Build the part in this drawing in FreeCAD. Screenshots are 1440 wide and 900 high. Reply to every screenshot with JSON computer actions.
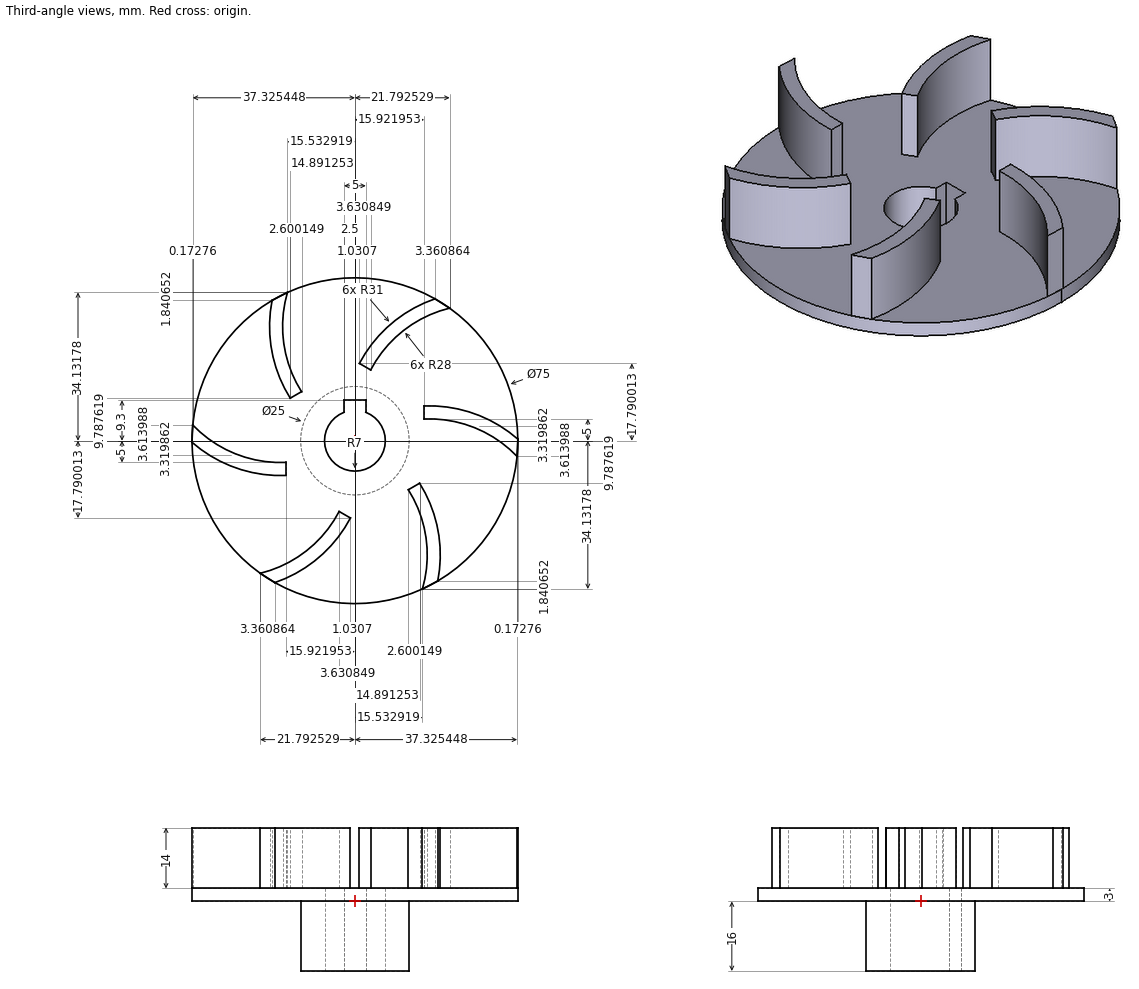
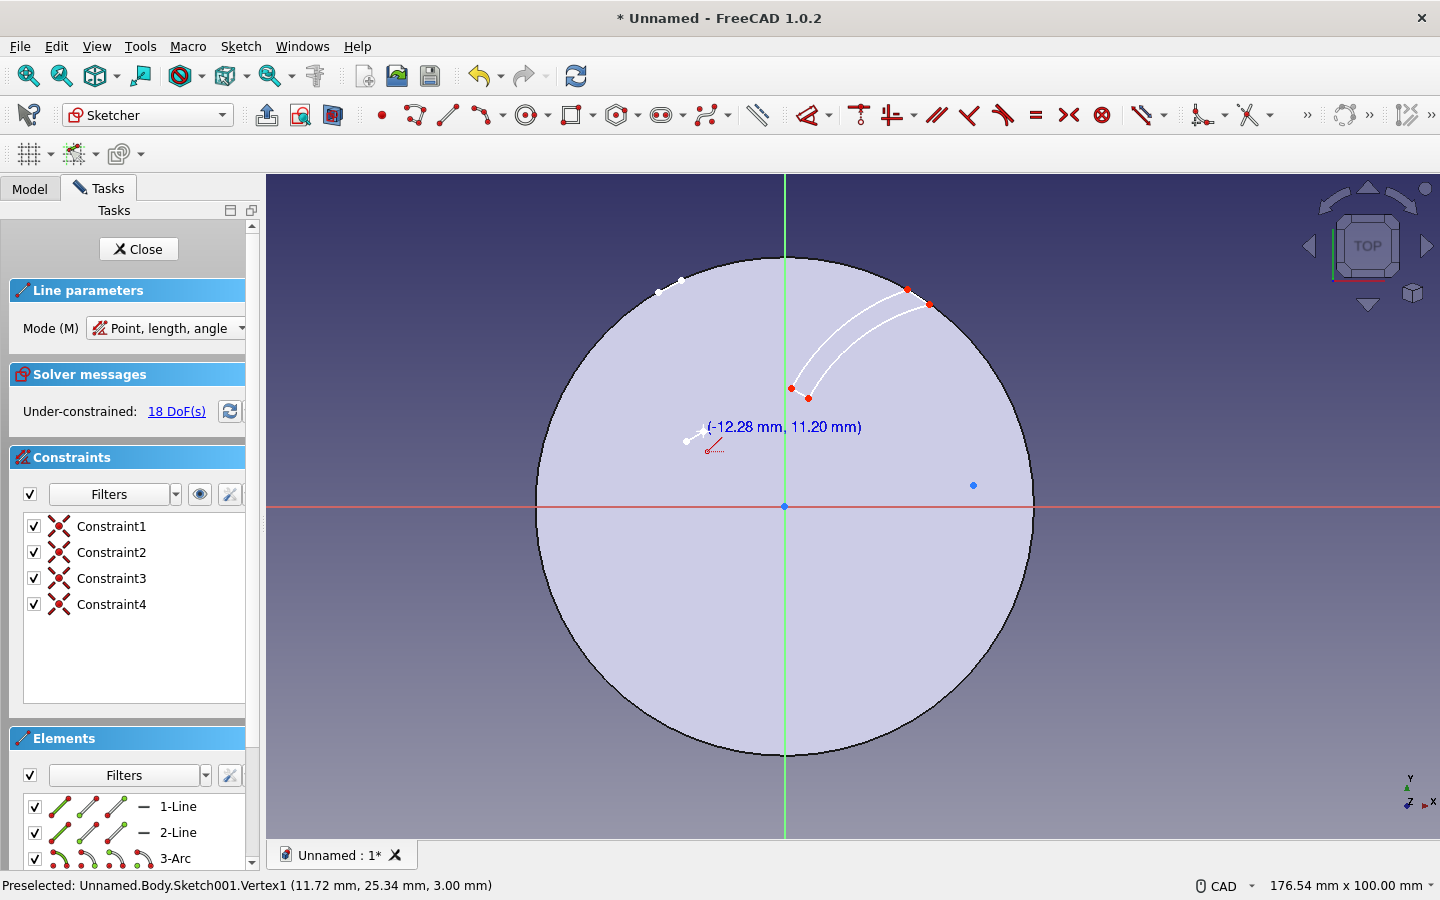
{"action": "left_click", "coordinate": [480, 116]}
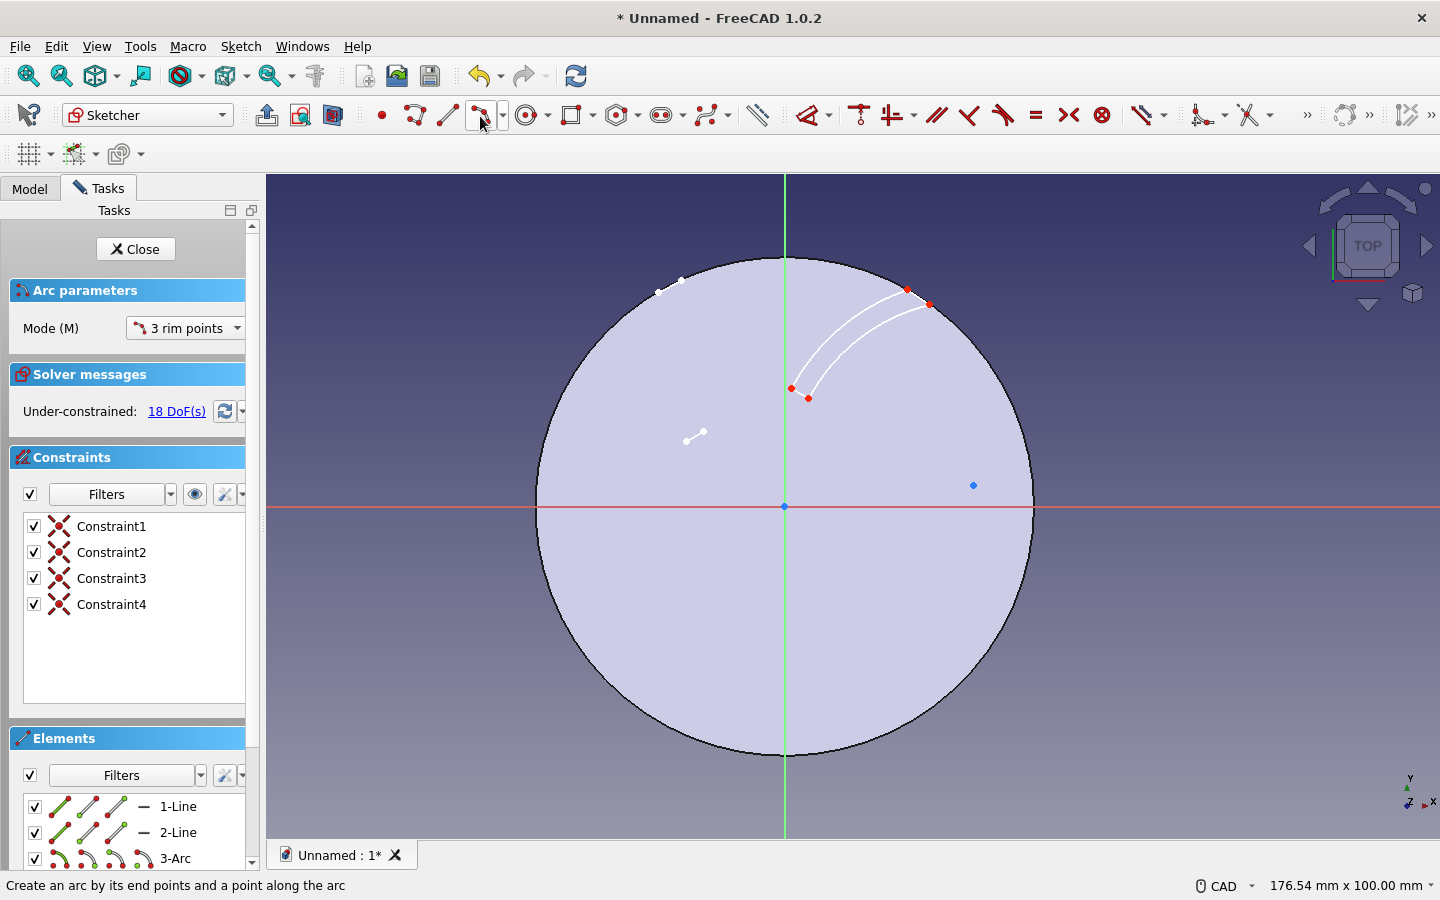
{"action": "left_click", "coordinate": [658, 293]}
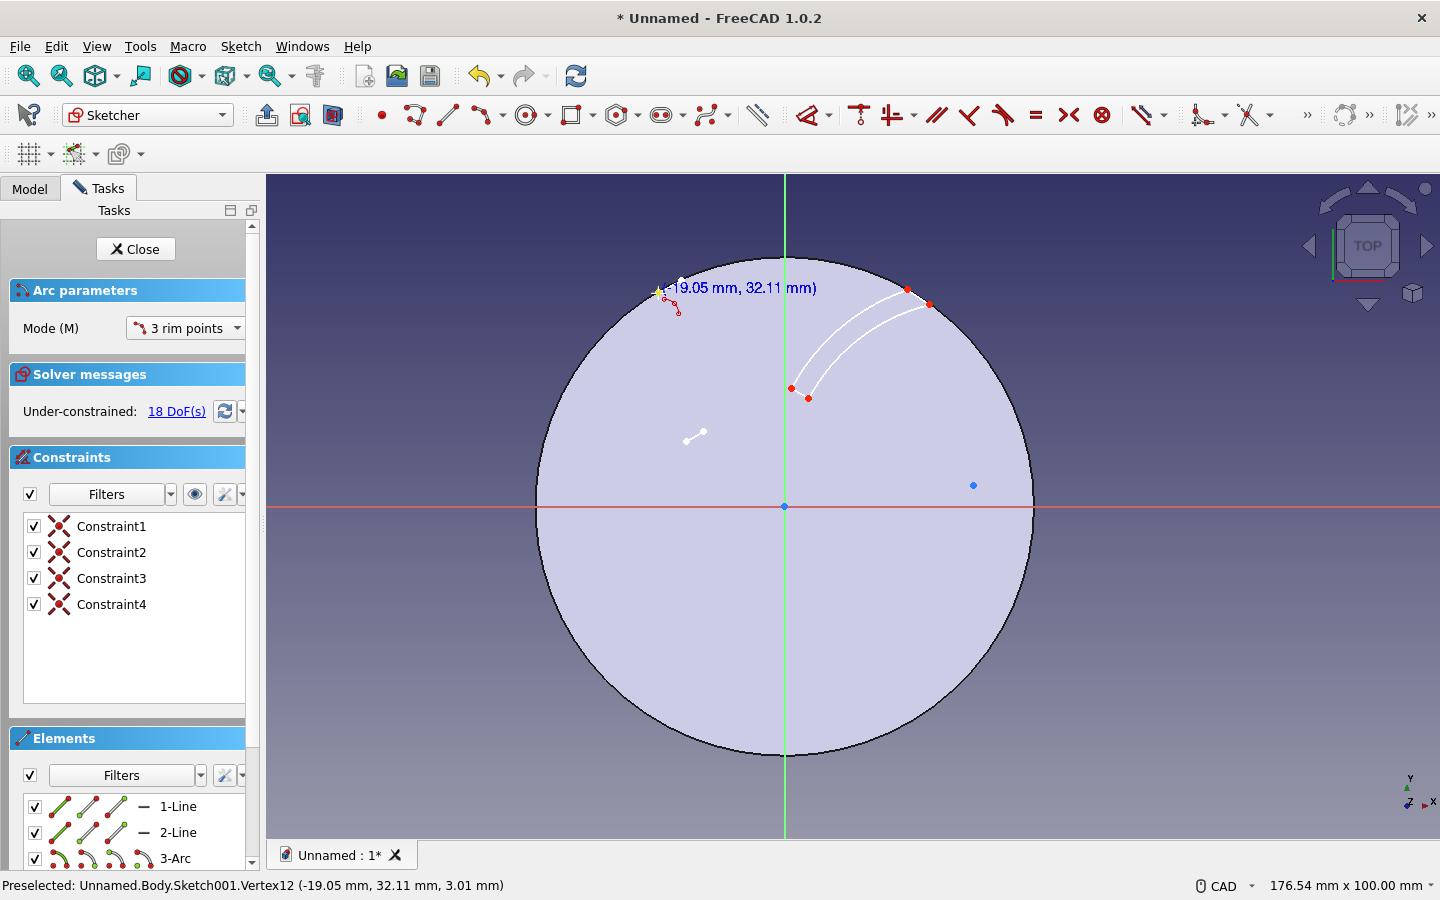
{"action": "scroll", "coordinate": [686, 441], "scroll_direction": "up", "scroll_amount": 3}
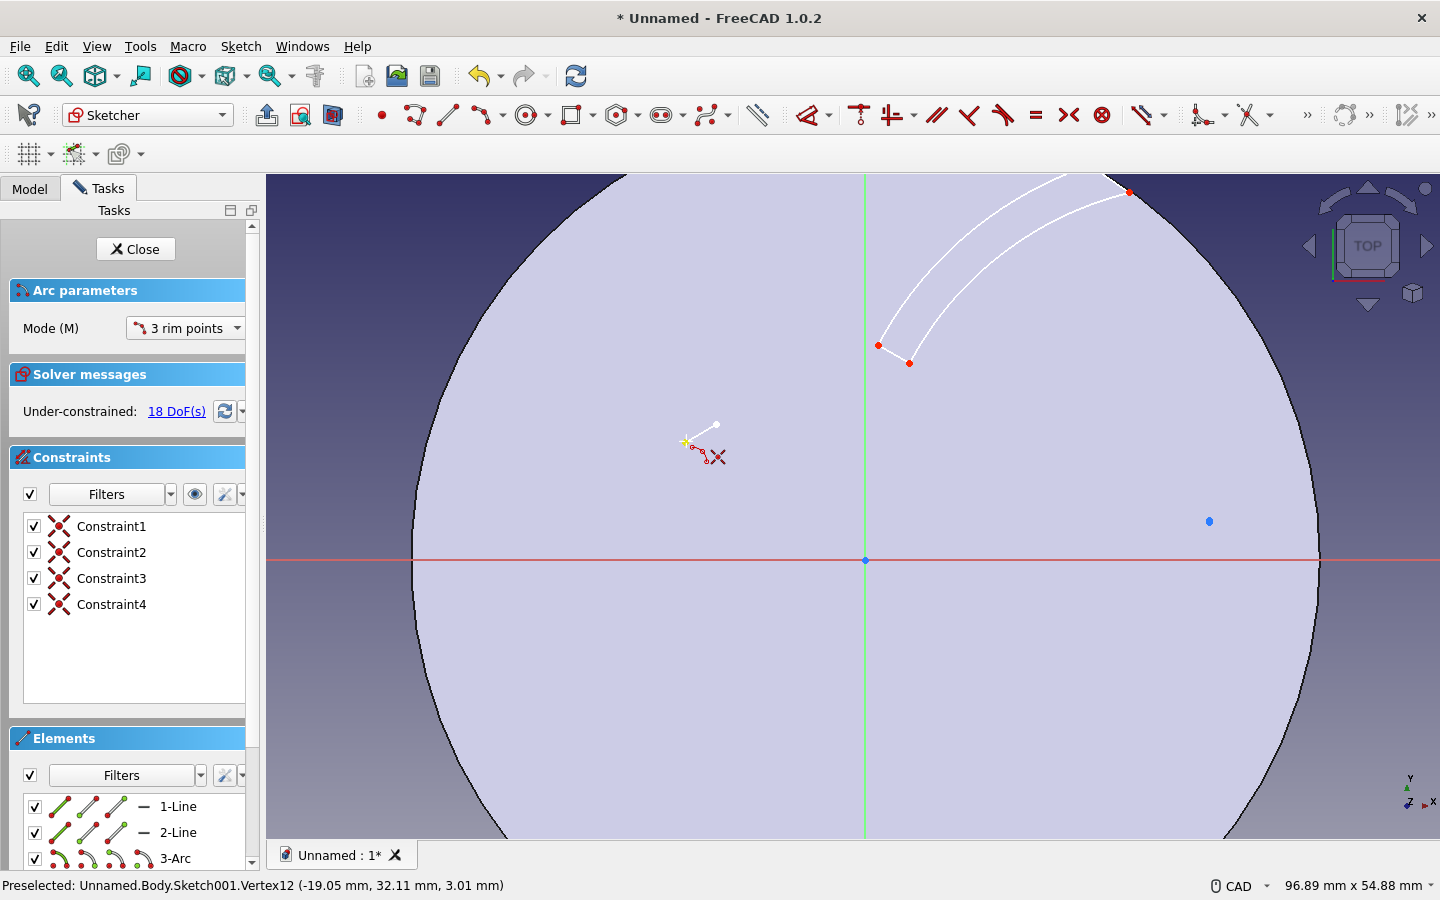
{"action": "left_click", "coordinate": [686, 442]}
{"action": "left_click", "coordinate": [634, 310]}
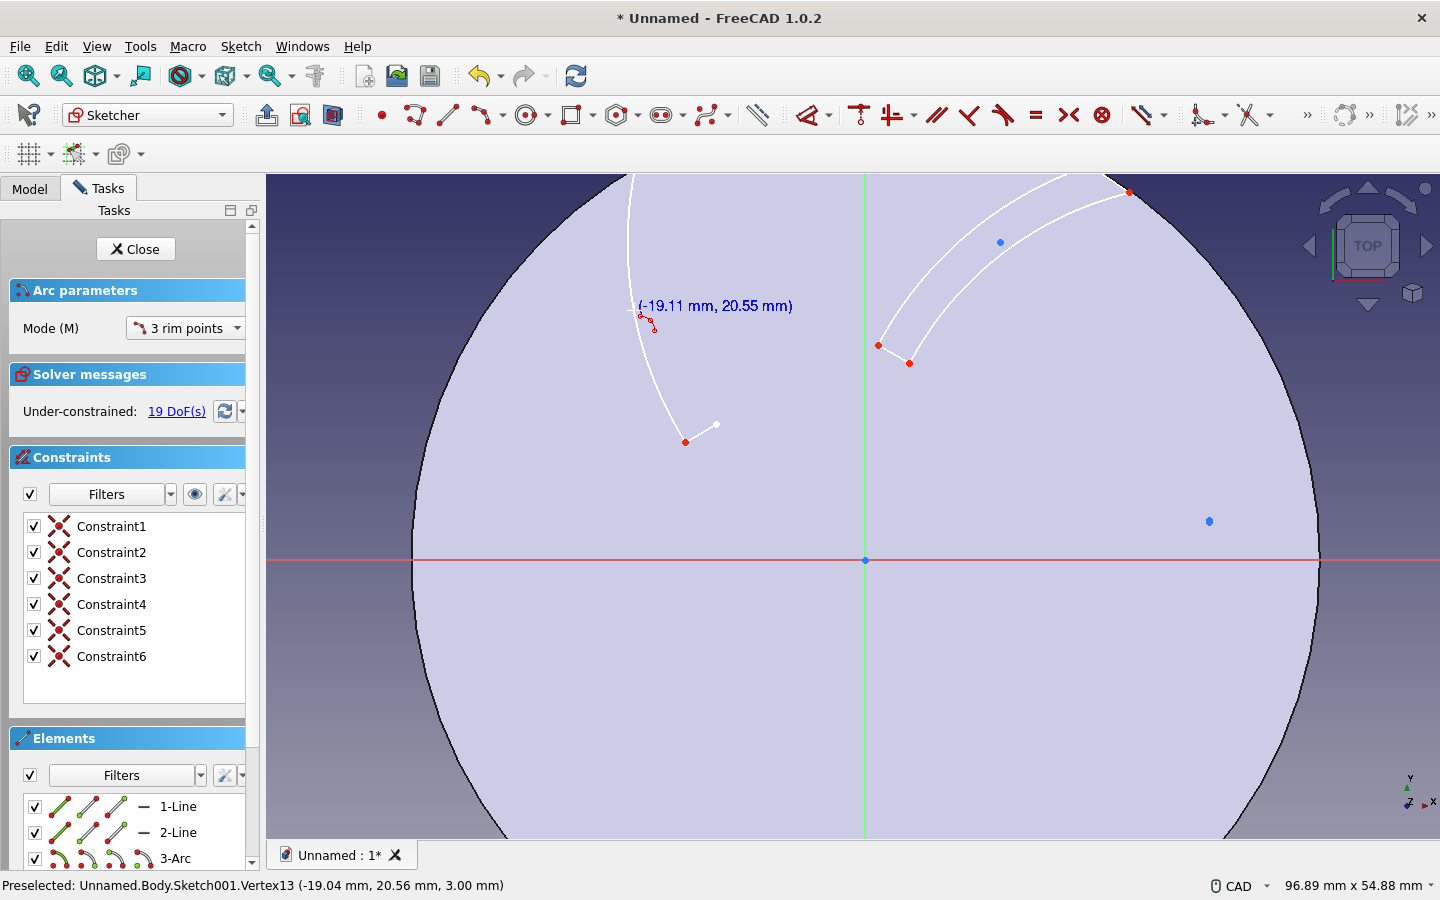
{"action": "left_click", "coordinate": [717, 424]}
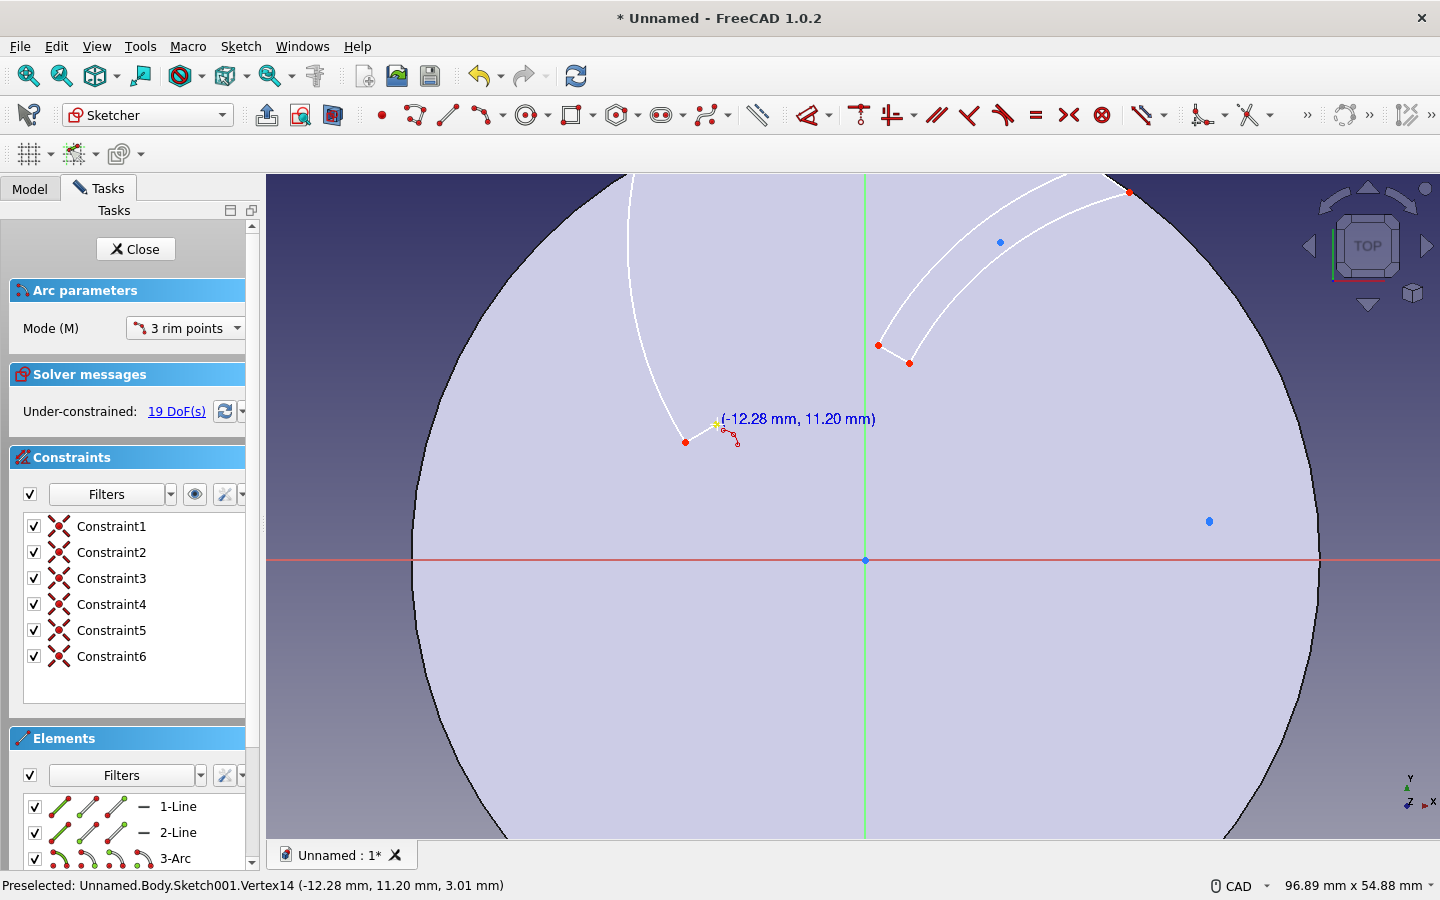
{"action": "scroll", "coordinate": [686, 441], "scroll_direction": "down", "scroll_amount": 3}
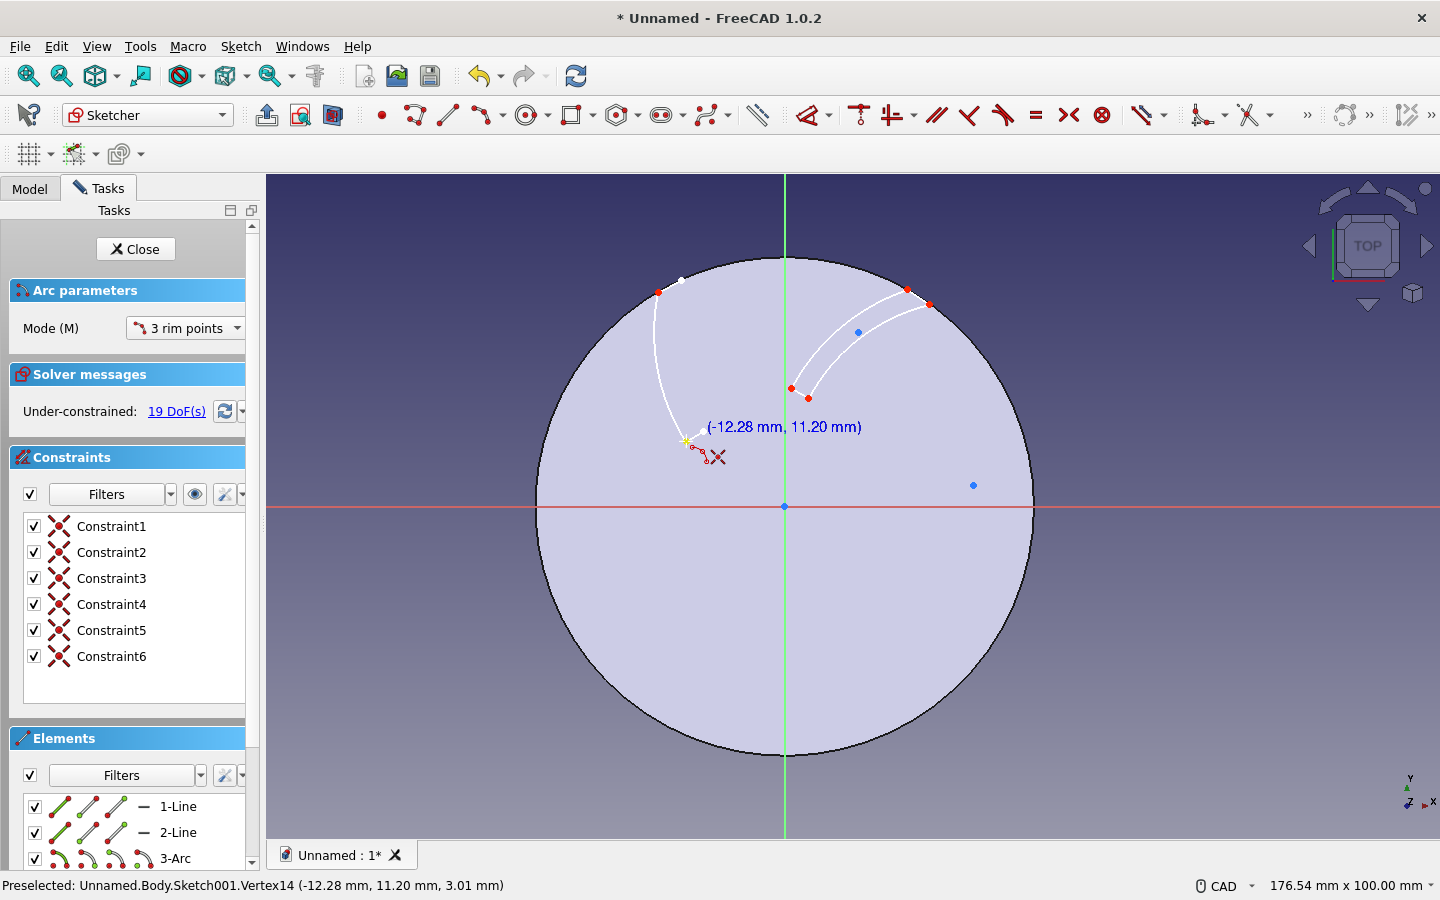
{"action": "left_click", "coordinate": [681, 281]}
{"action": "left_click", "coordinate": [676, 358]}